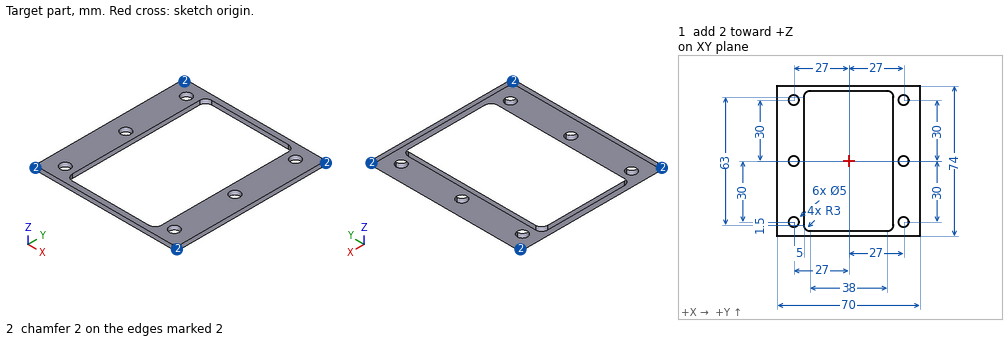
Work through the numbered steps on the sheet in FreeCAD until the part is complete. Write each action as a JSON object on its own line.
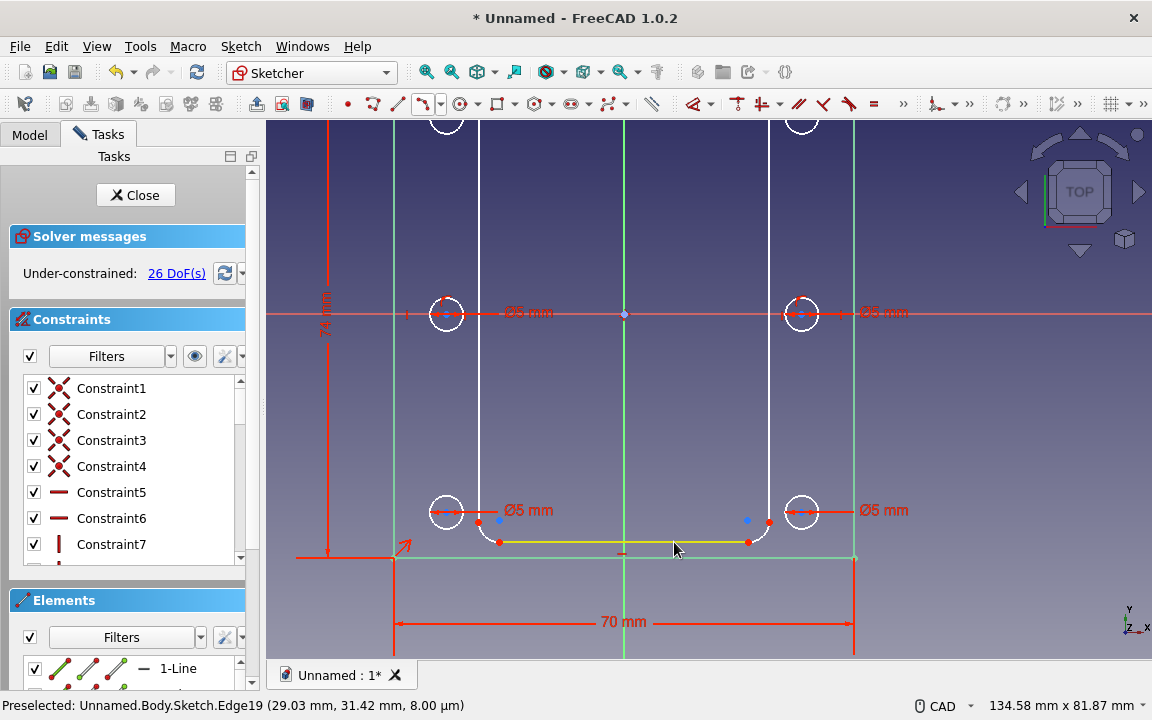
{"action": "left_click", "coordinate": [674, 542]}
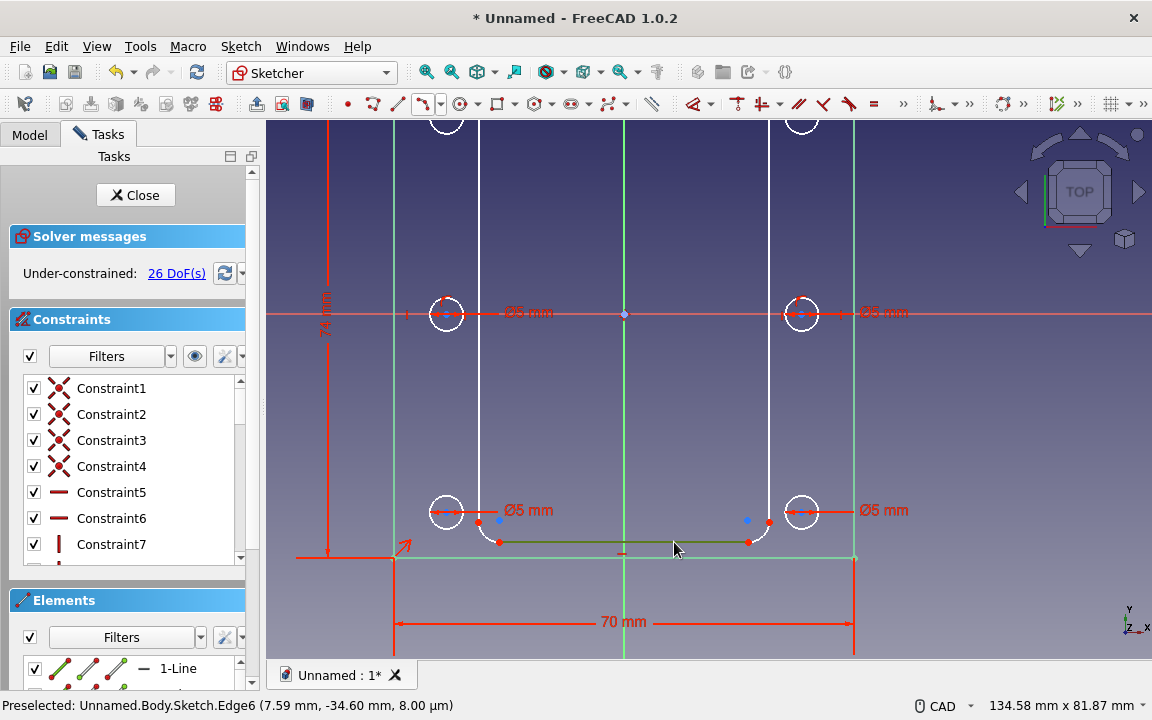
{"action": "scroll", "coordinate": [481, 532], "scroll_direction": "up", "scroll_amount": 2}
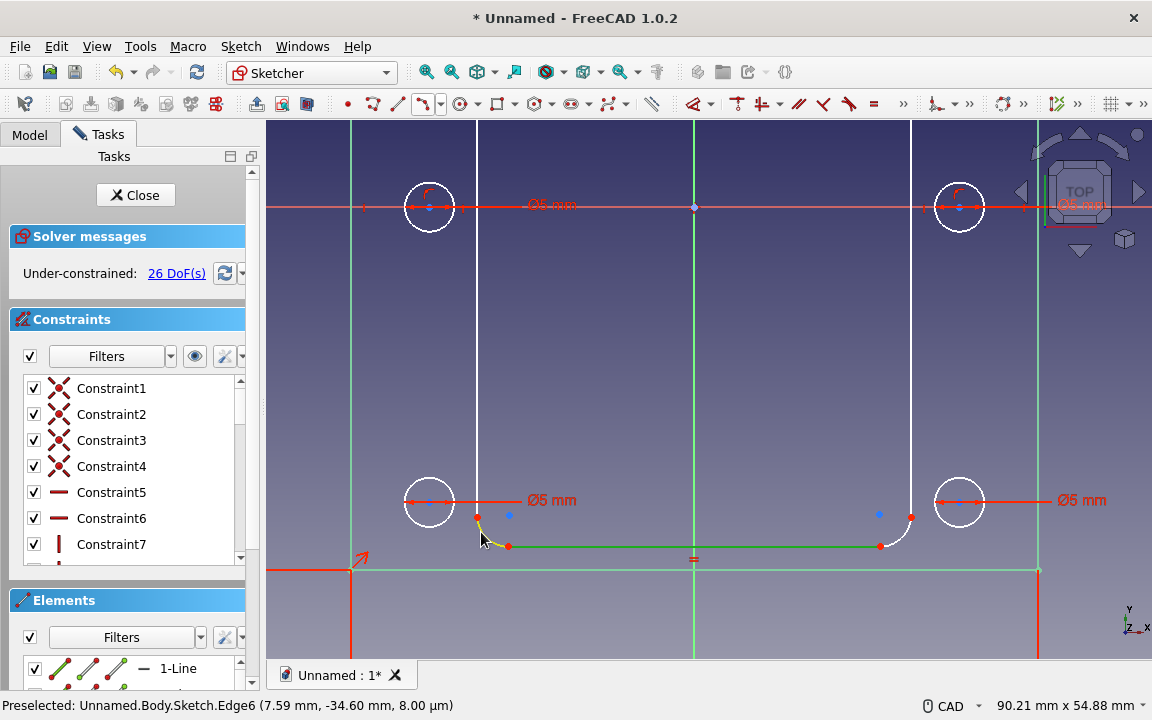
{"action": "left_click", "coordinate": [482, 531]}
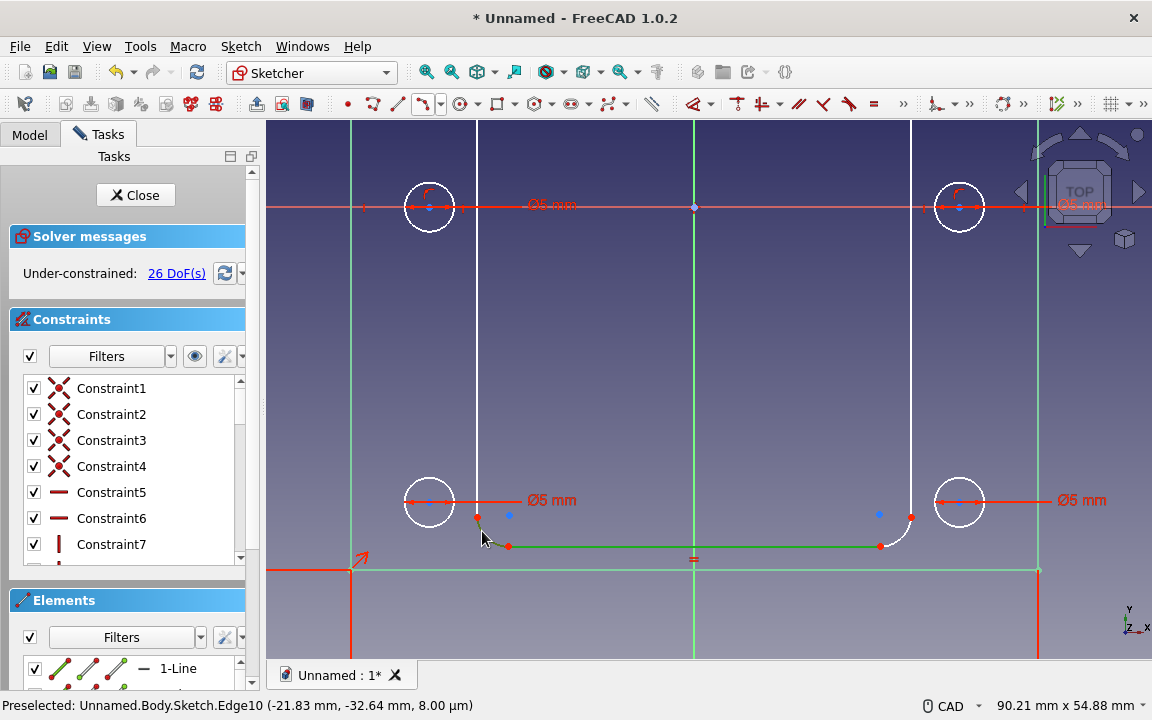
{"action": "left_click", "coordinate": [849, 104]}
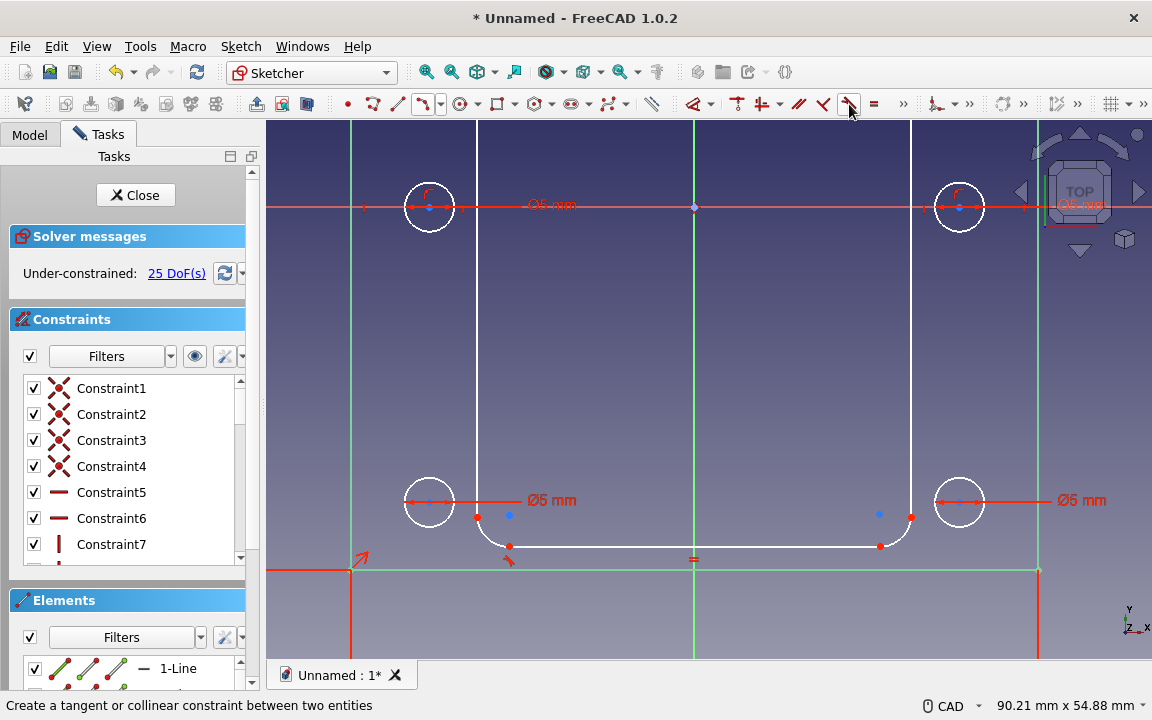
{"action": "left_click", "coordinate": [769, 547]}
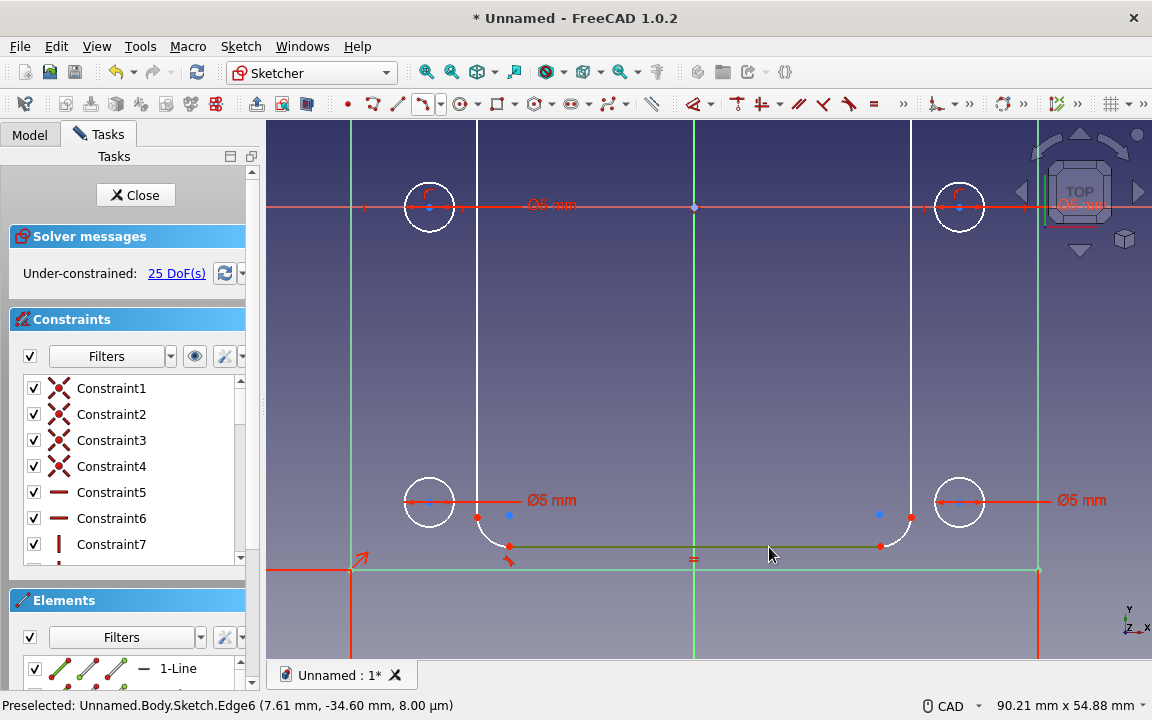
{"action": "left_click", "coordinate": [894, 544]}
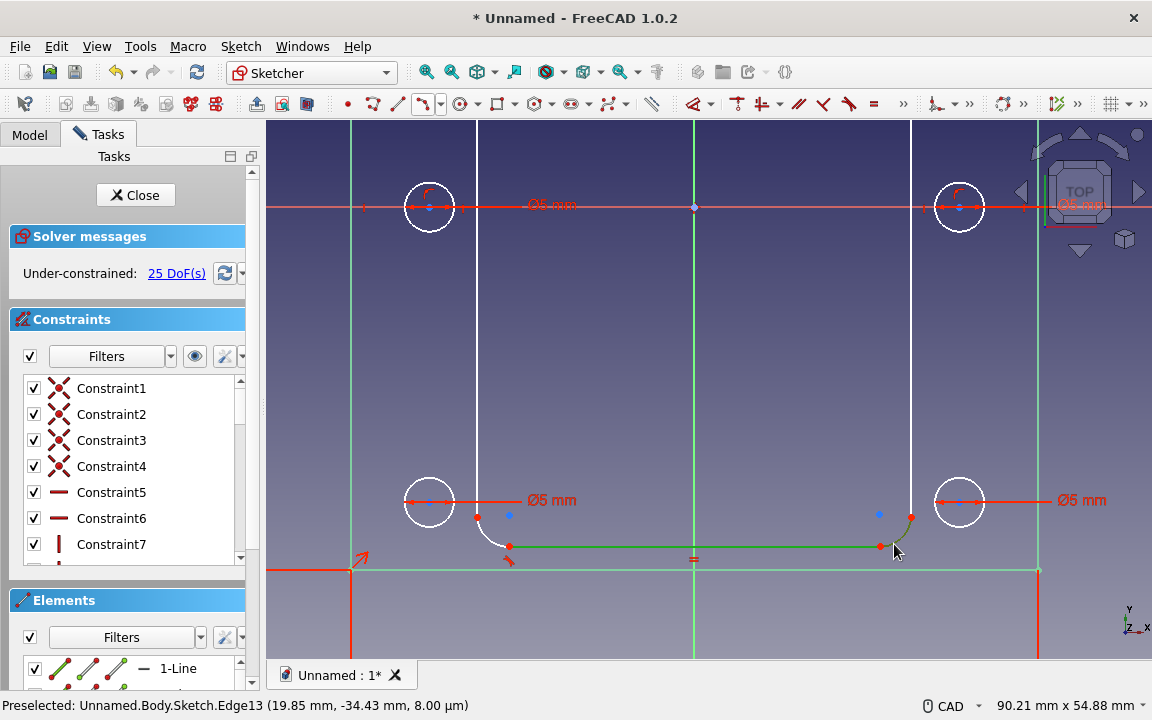
{"action": "left_click", "coordinate": [849, 104]}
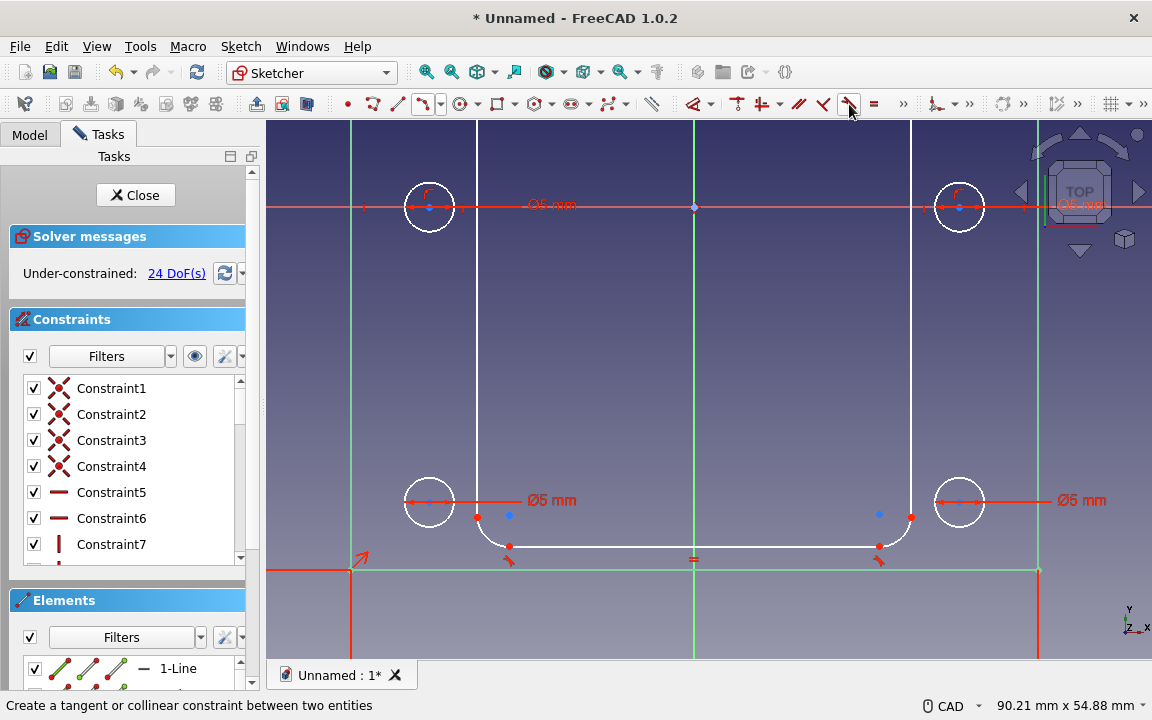
{"action": "left_click", "coordinate": [477, 332]}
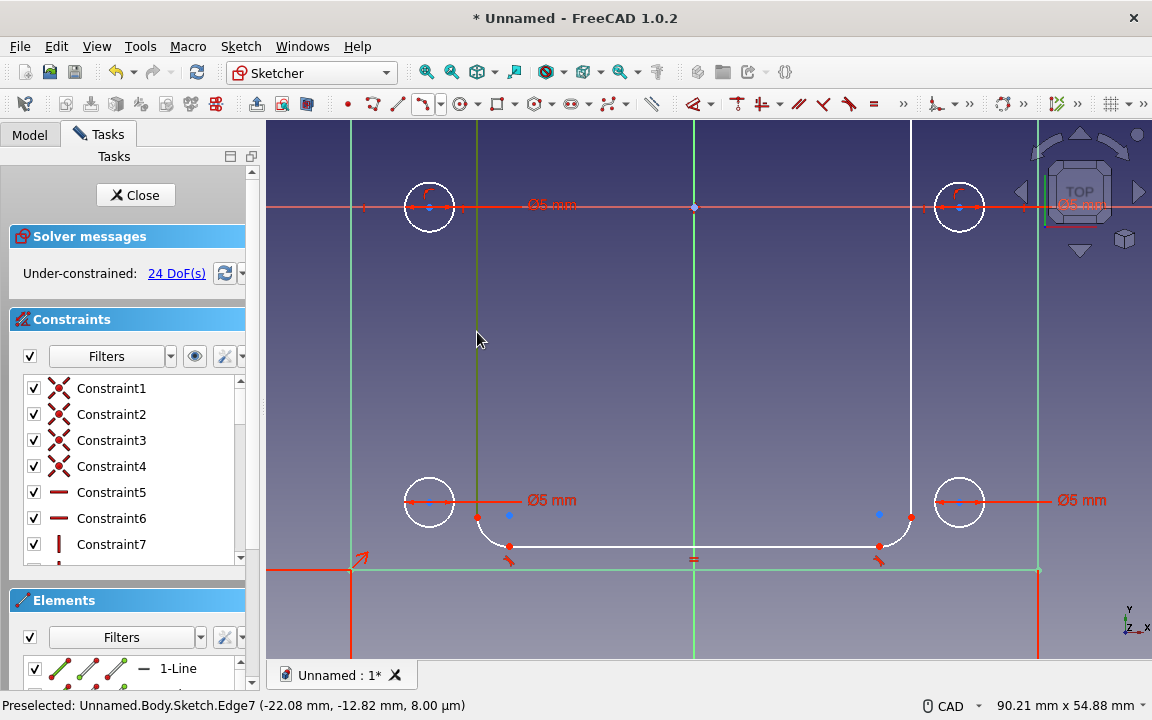
{"action": "left_click", "coordinate": [482, 531]}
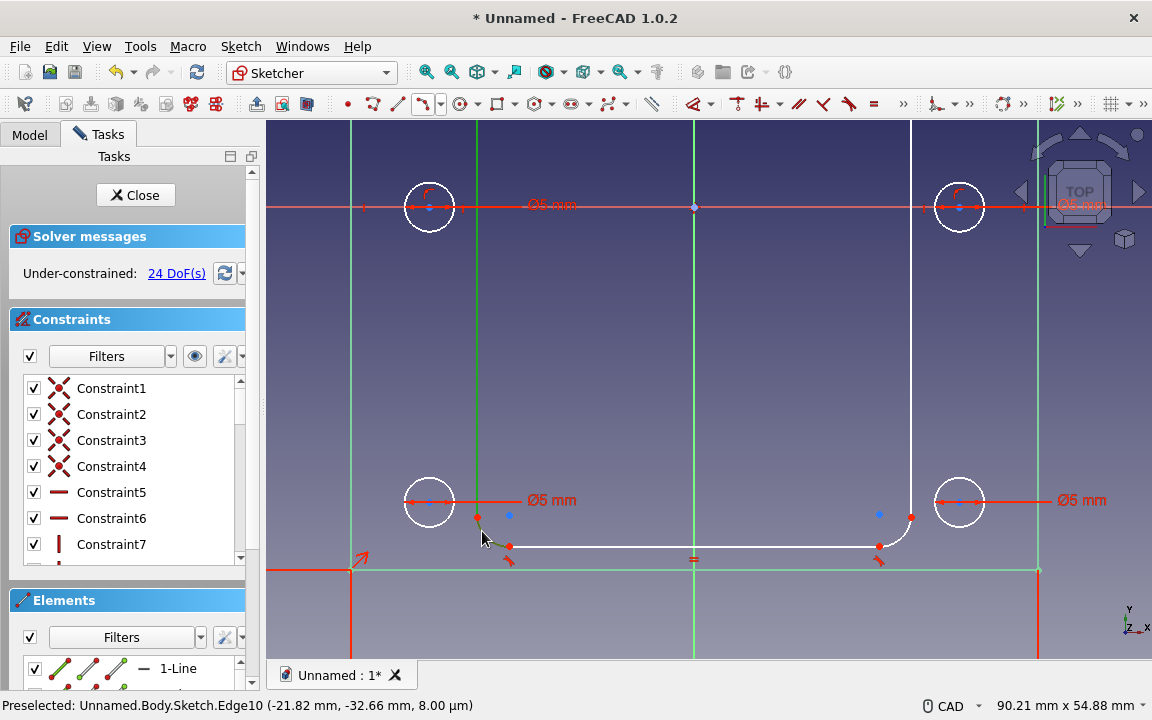
{"action": "left_click", "coordinate": [849, 104]}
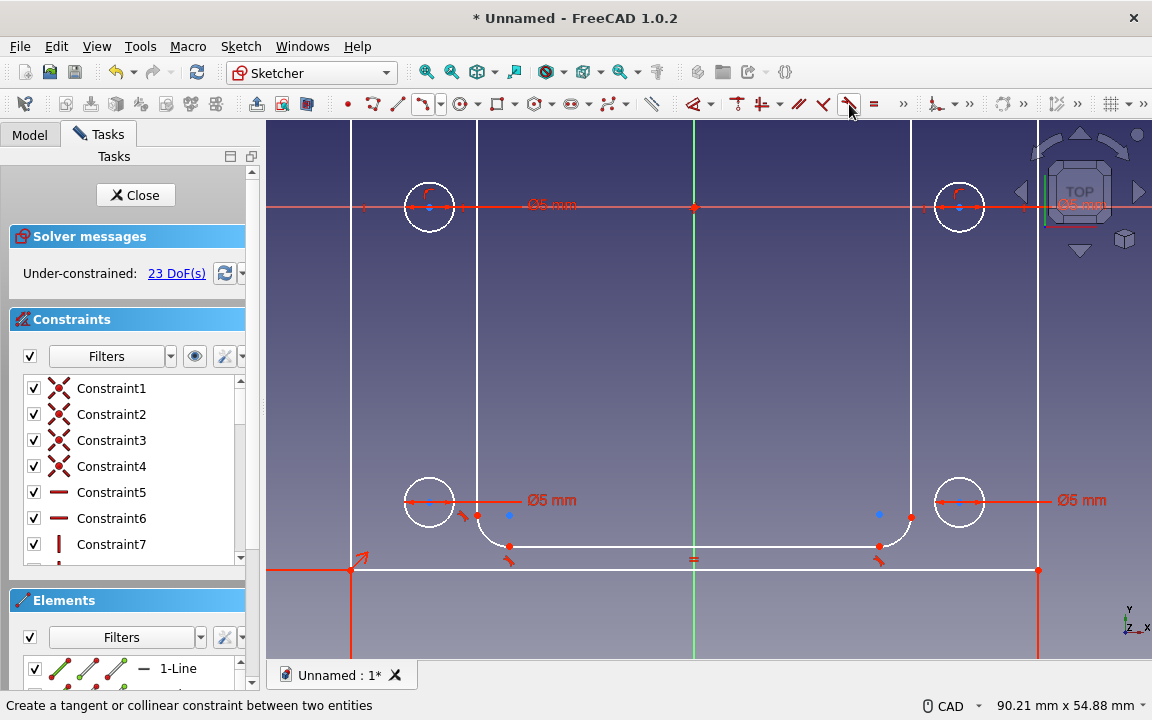
{"action": "left_click", "coordinate": [477, 331]}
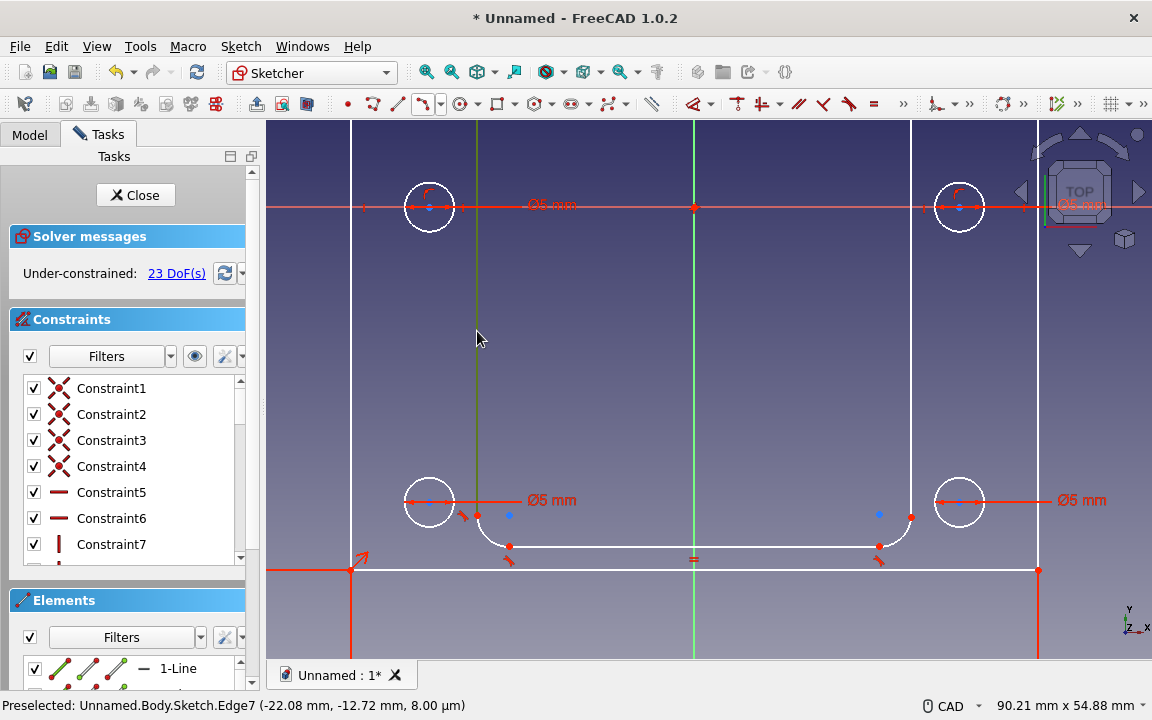
{"action": "scroll", "coordinate": [597, 538], "scroll_direction": "down", "scroll_amount": 4}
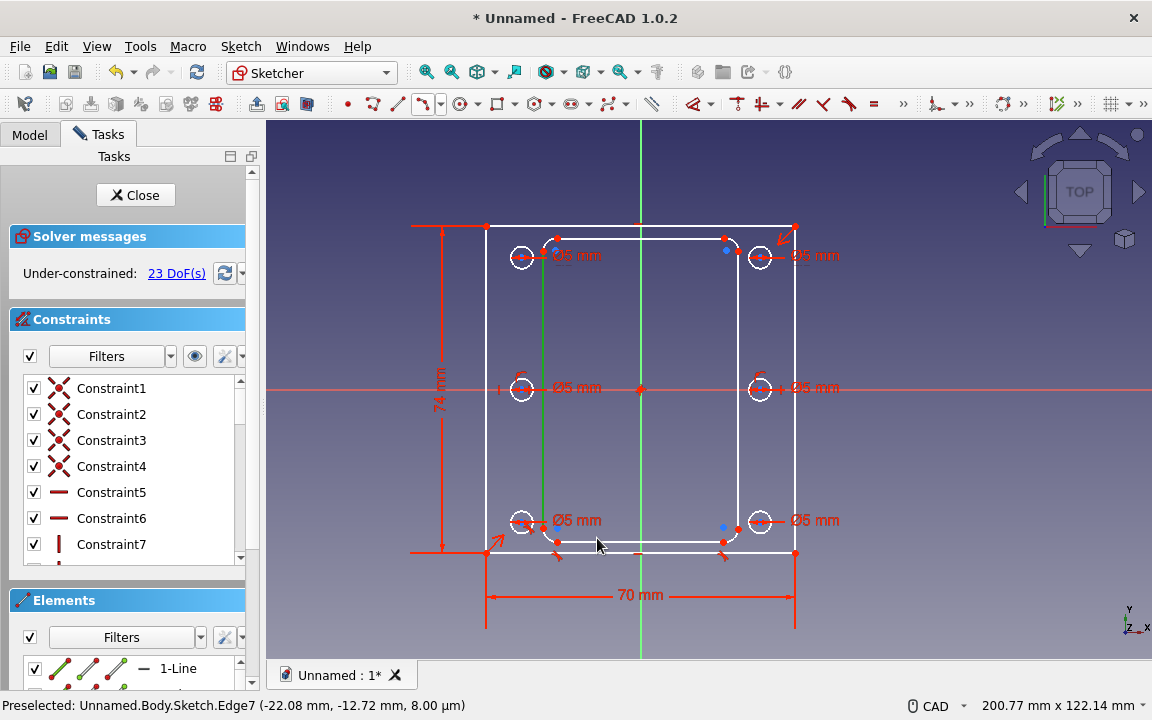
{"action": "scroll", "coordinate": [551, 239], "scroll_direction": "up", "scroll_amount": 4}